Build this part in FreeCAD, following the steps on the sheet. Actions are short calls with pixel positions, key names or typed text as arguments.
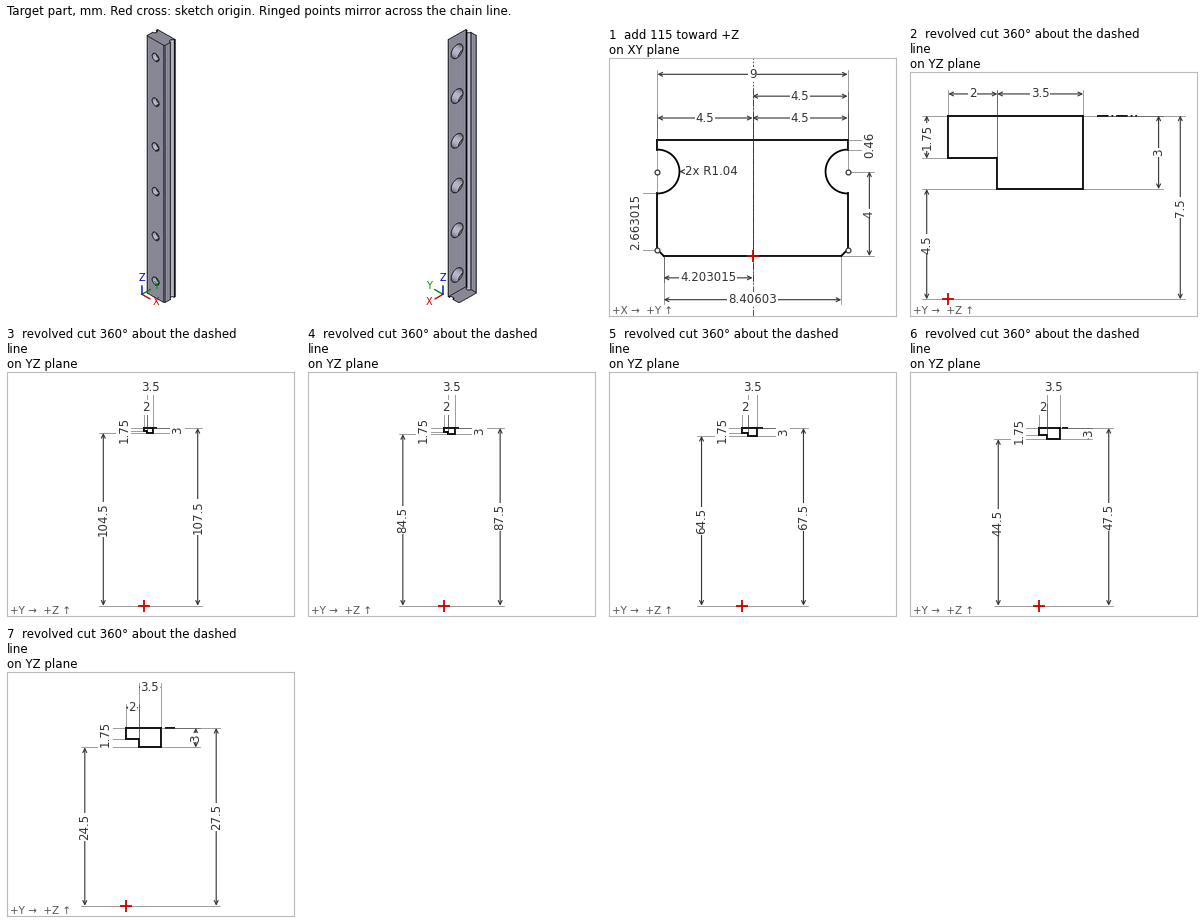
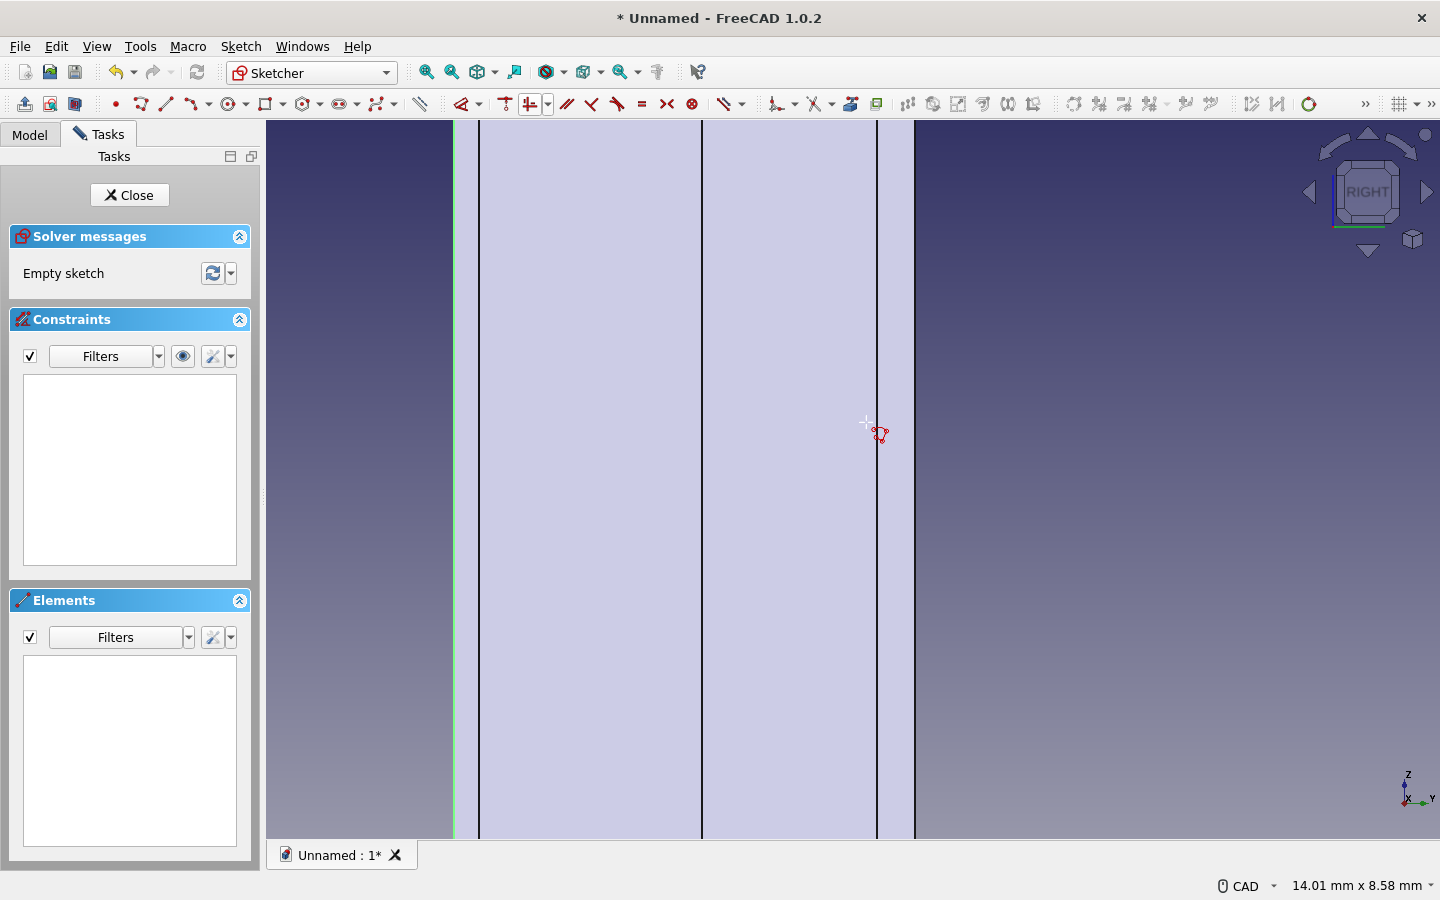
click(622, 604)
click(915, 604)
click(915, 353)
click(454, 353)
click(463, 499)
click(622, 499)
click(622, 605)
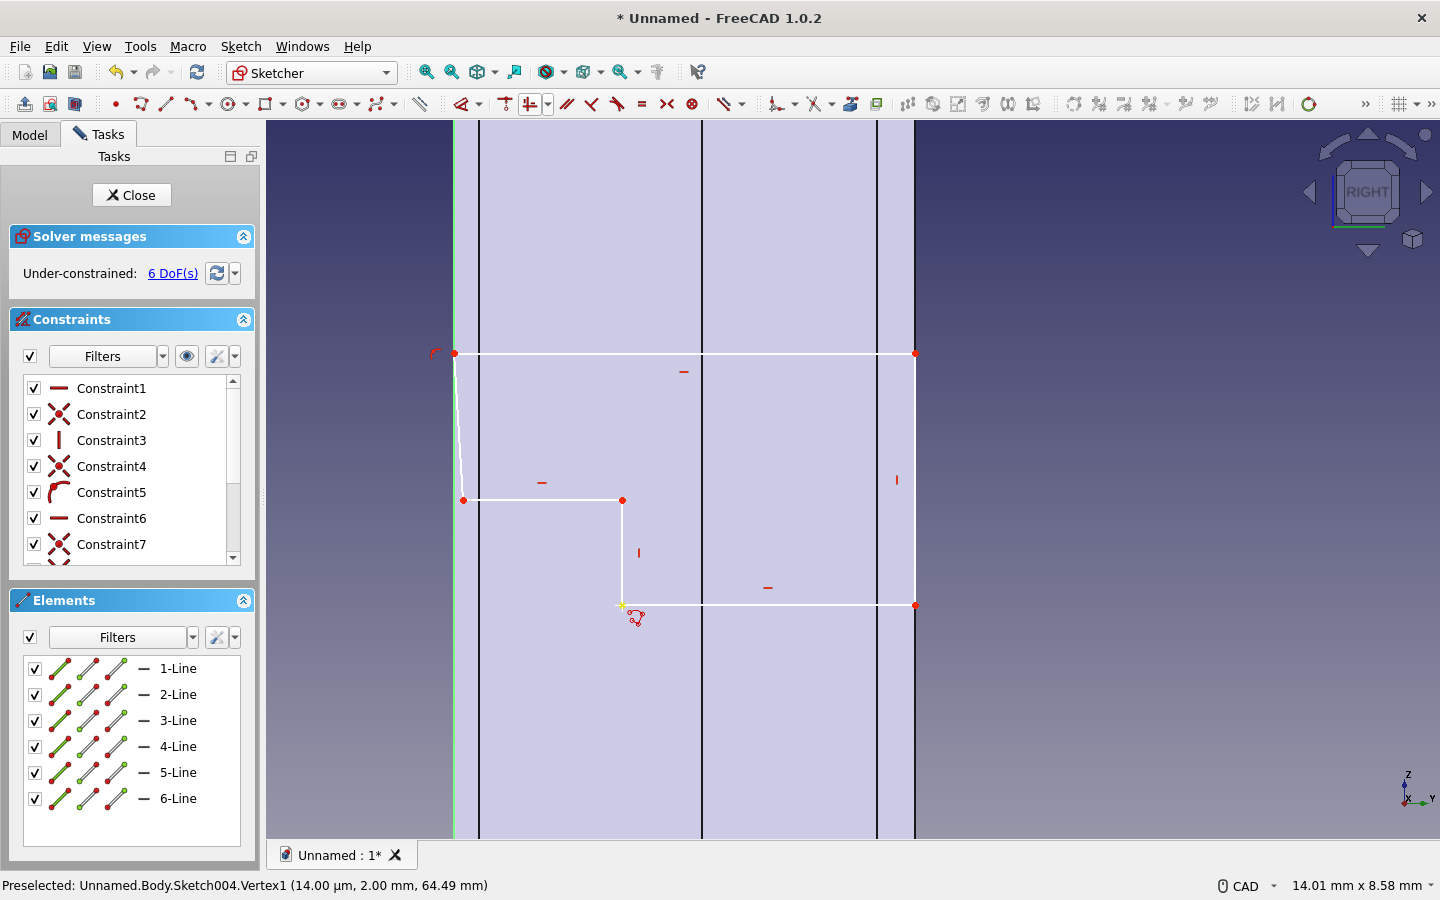
key(g)
key(l)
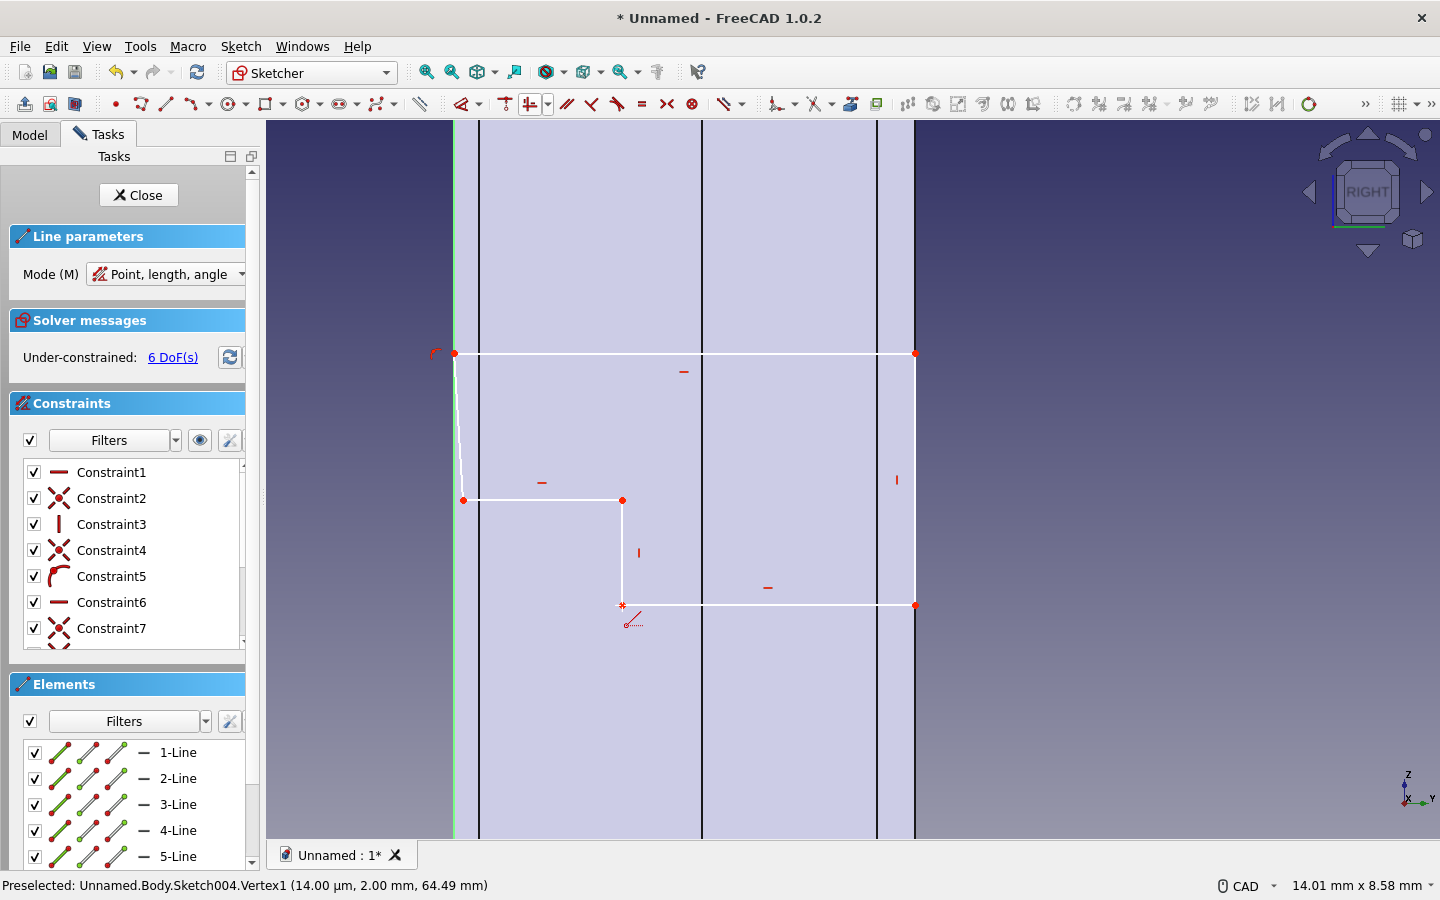
click(961, 353)
click(1100, 353)
key(Escape)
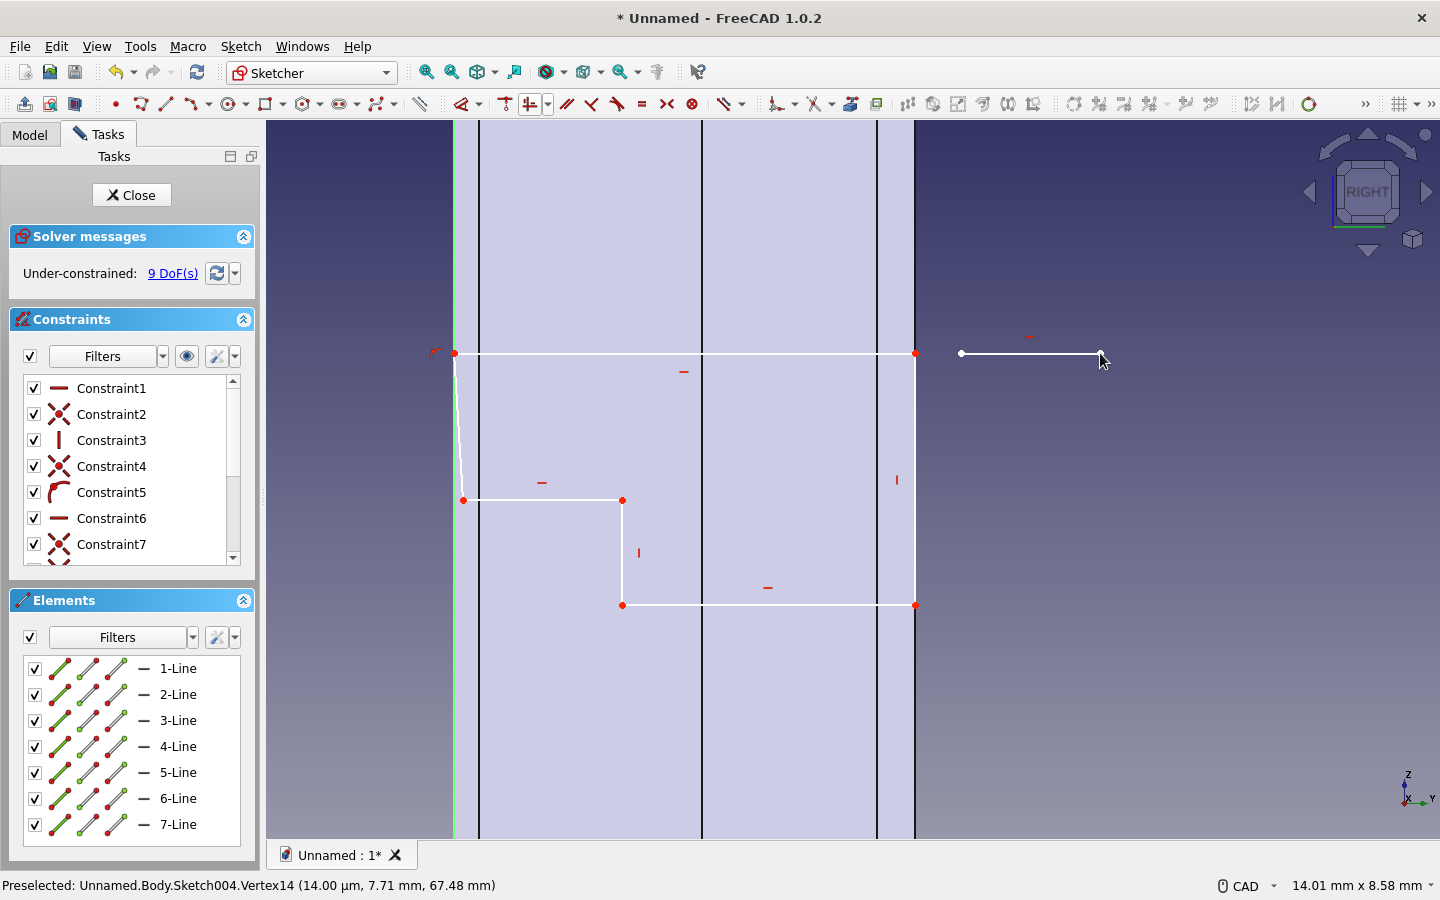
click(1003, 354)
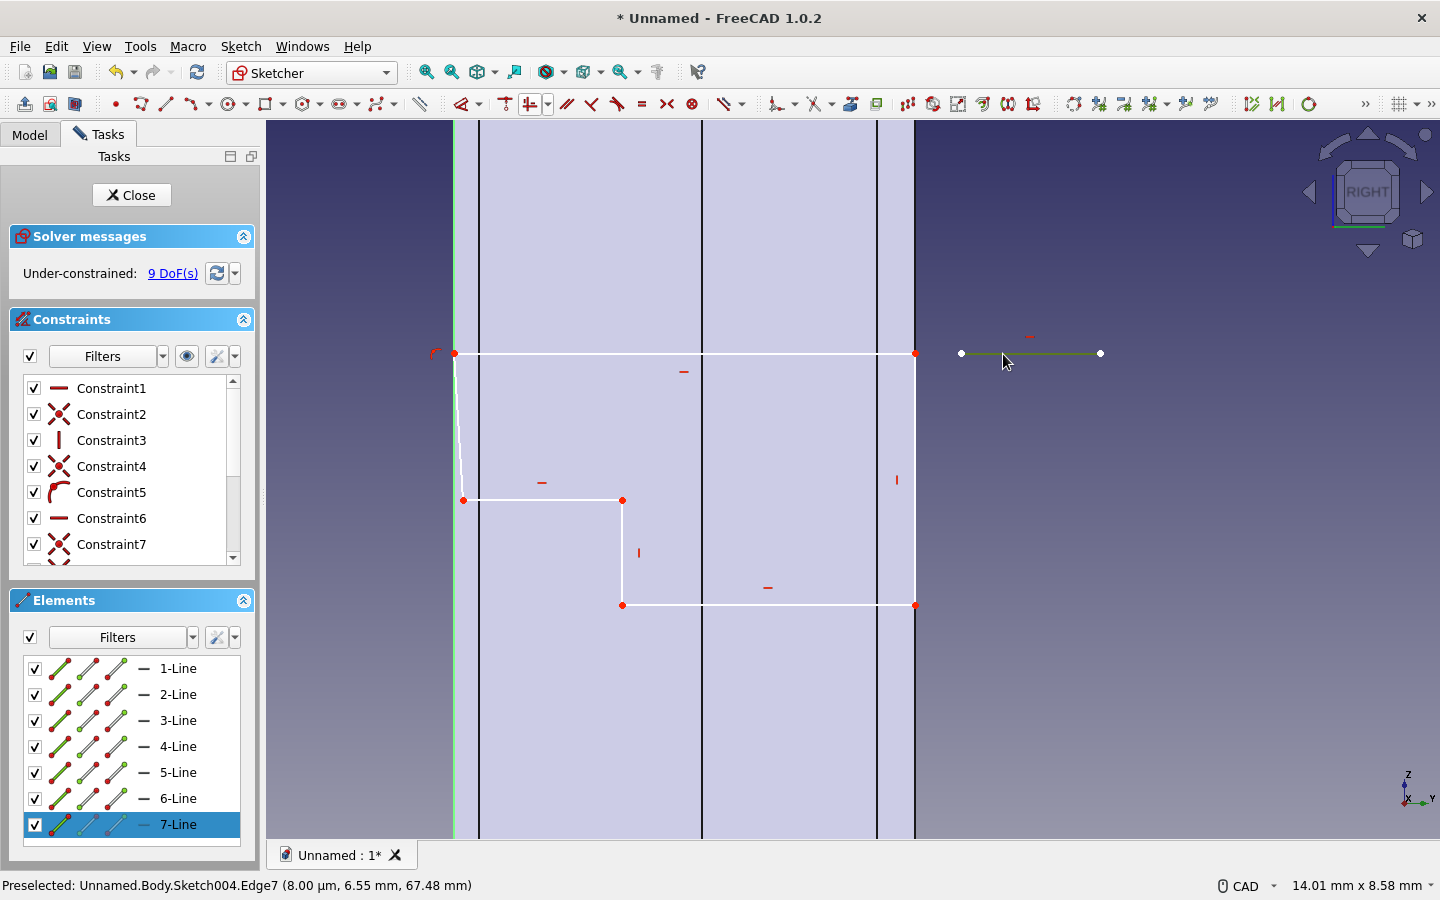
key(g)
key(n)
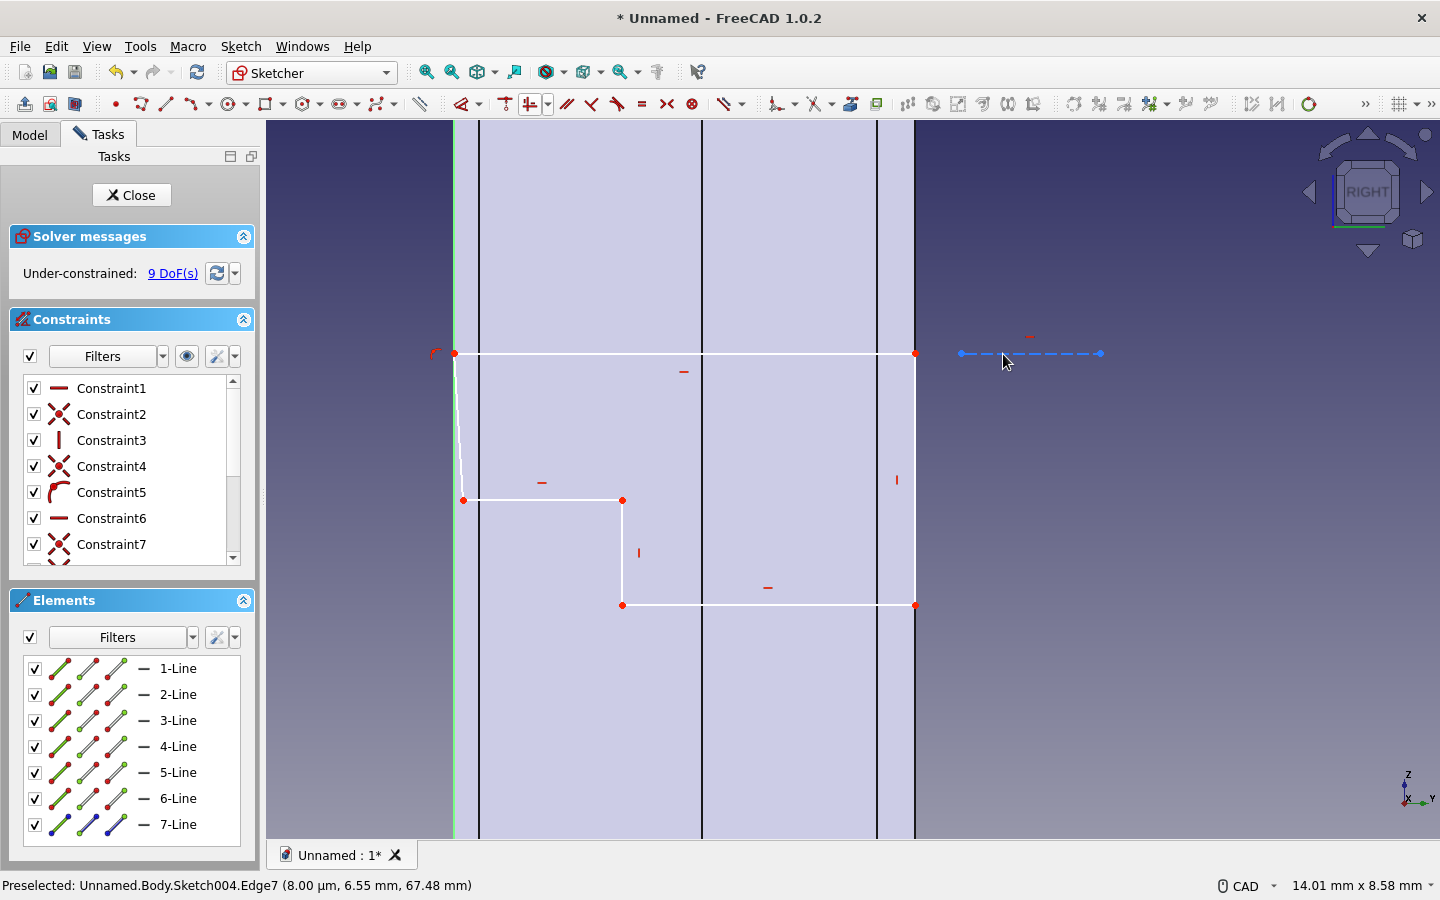
click(457, 398)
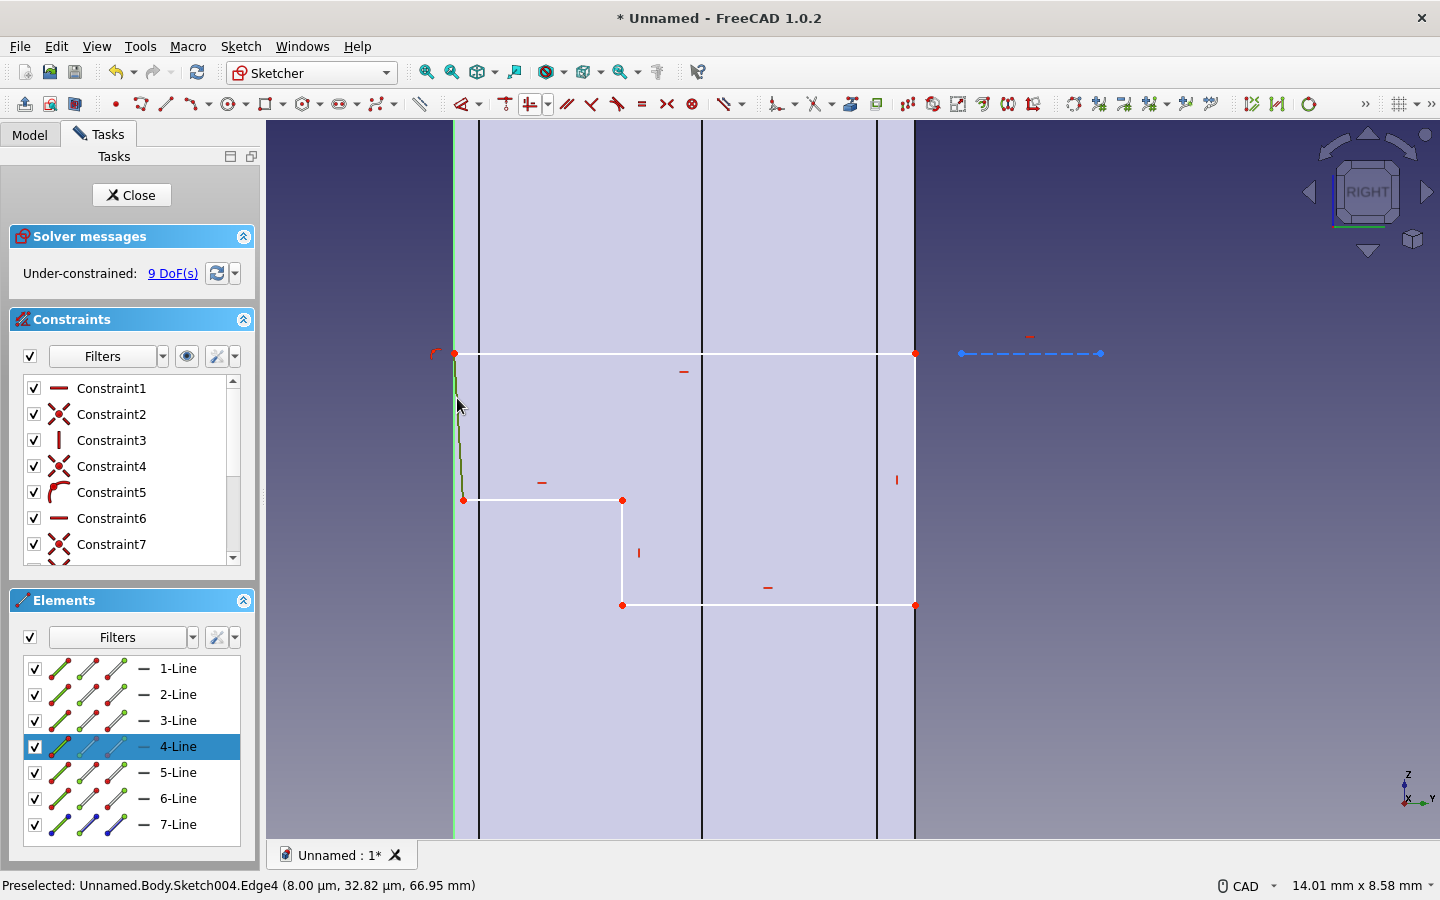
key(v)